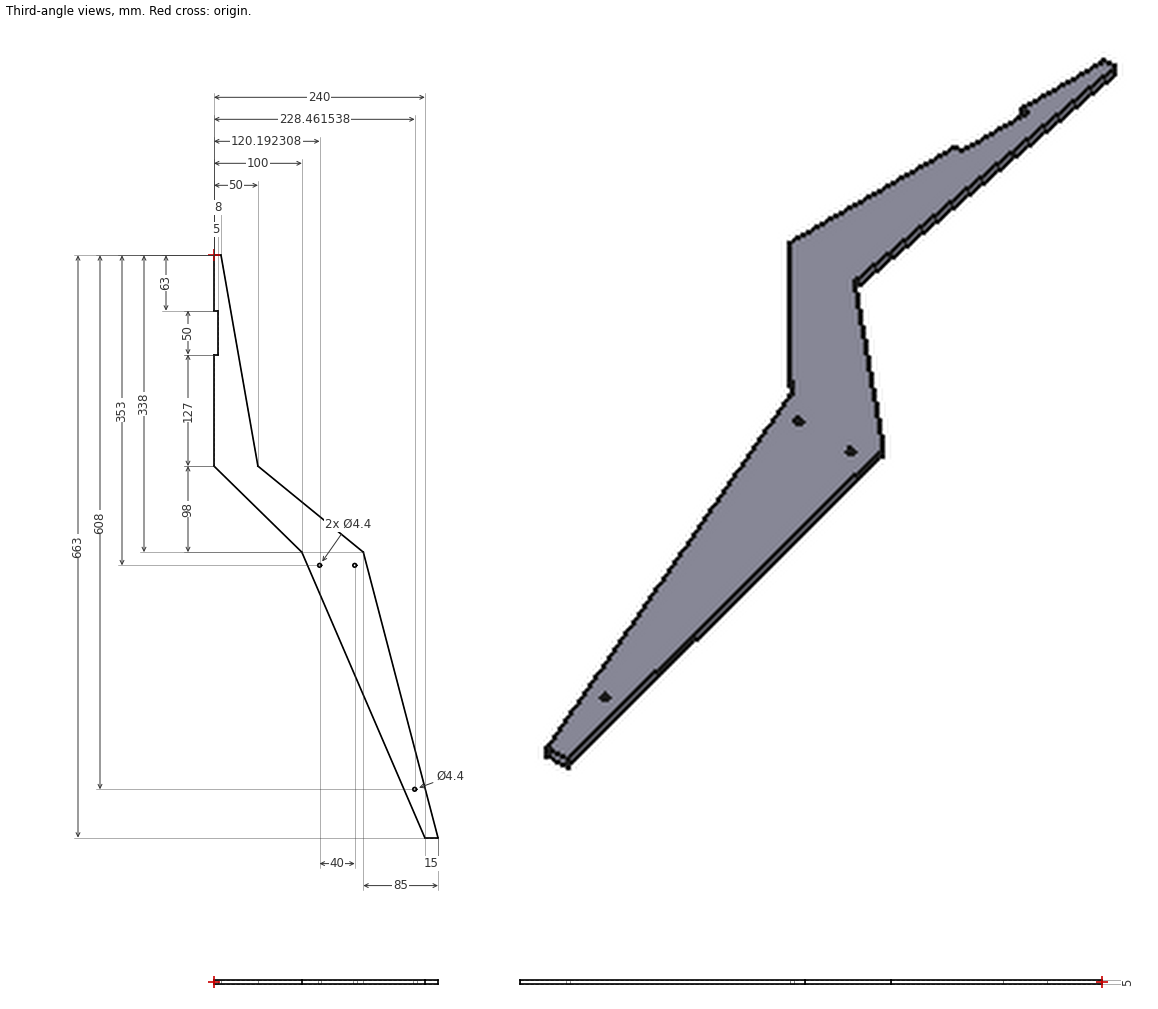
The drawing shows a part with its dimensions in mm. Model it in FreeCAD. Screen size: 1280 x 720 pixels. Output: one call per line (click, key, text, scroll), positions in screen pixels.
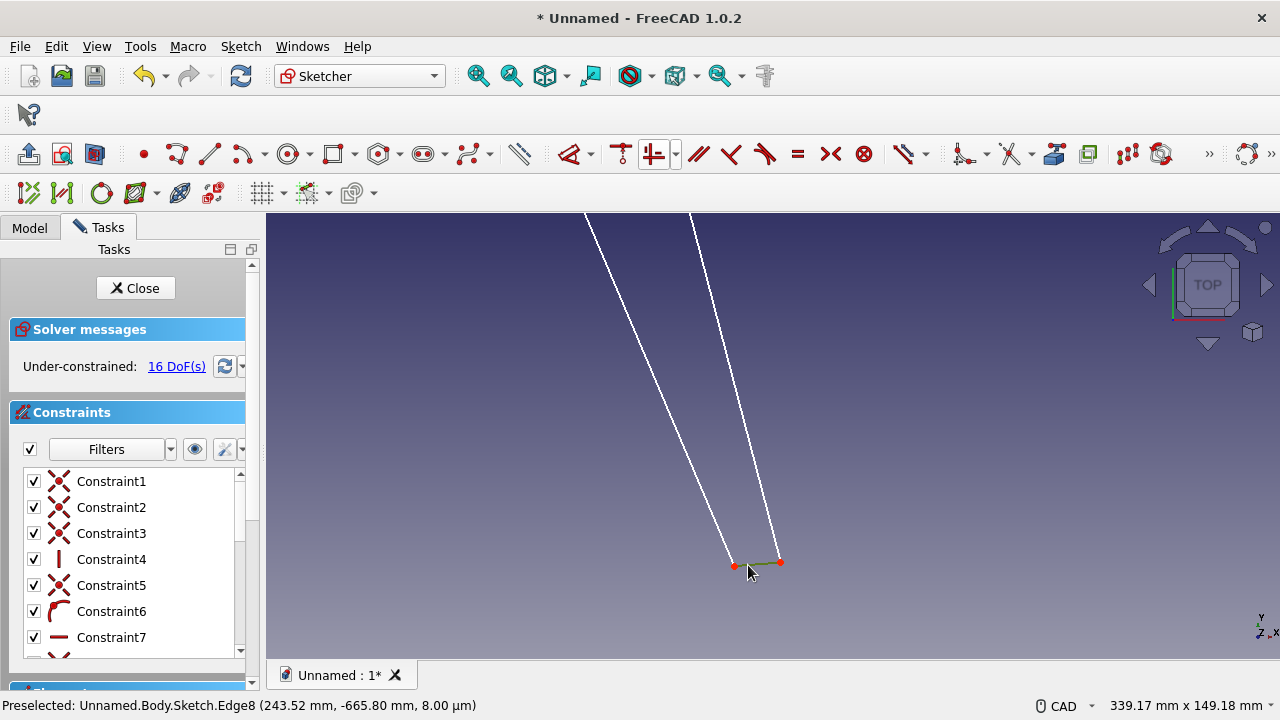
key(h)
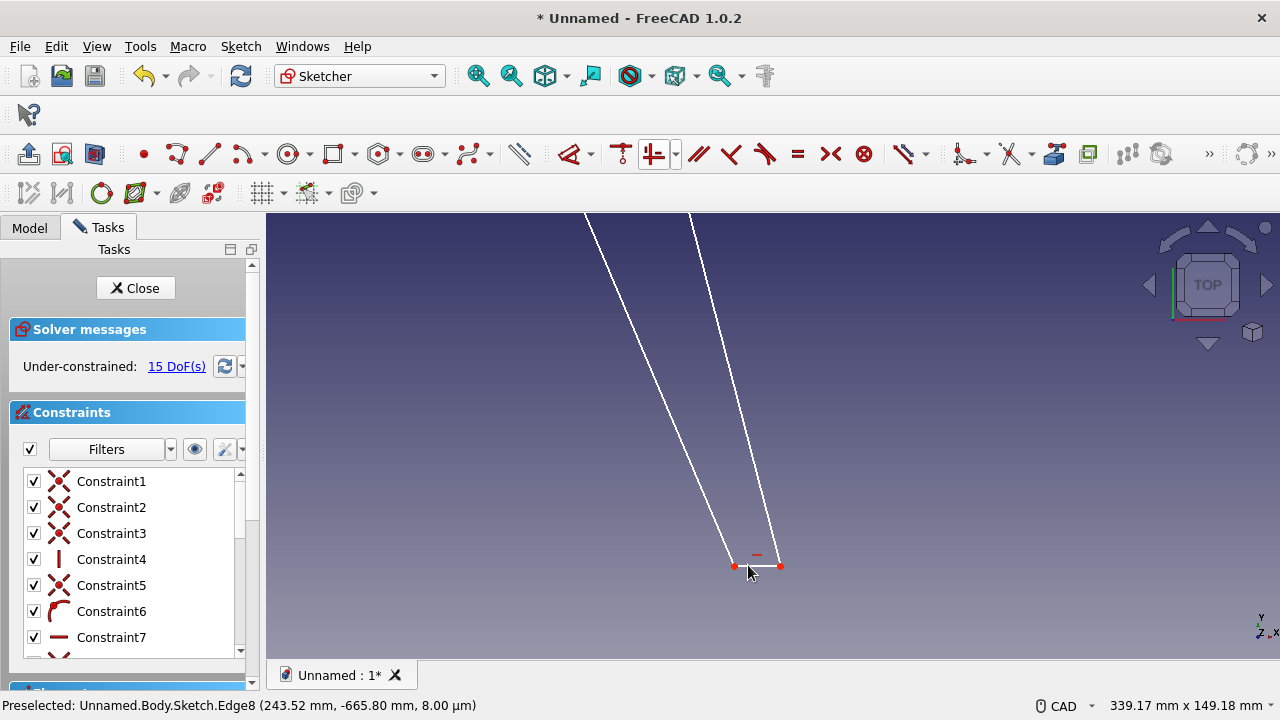
scroll(752, 572, down, 10)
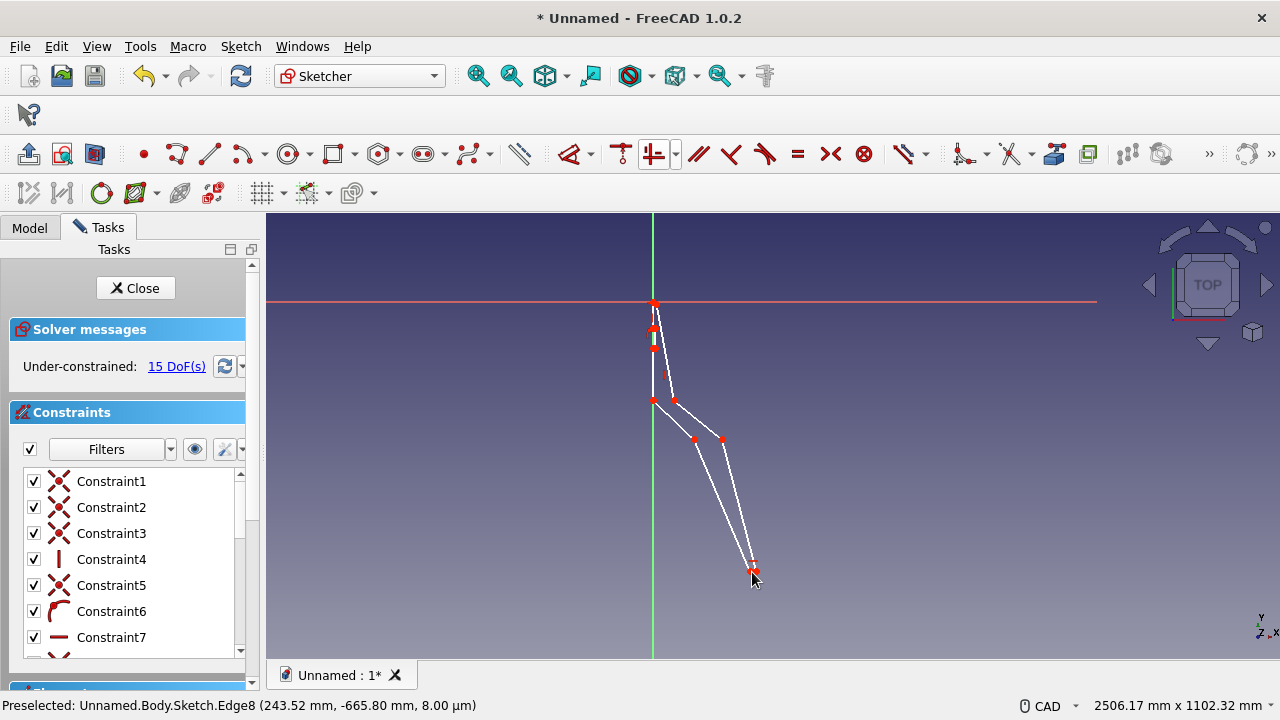
scroll(655, 304, up, 12)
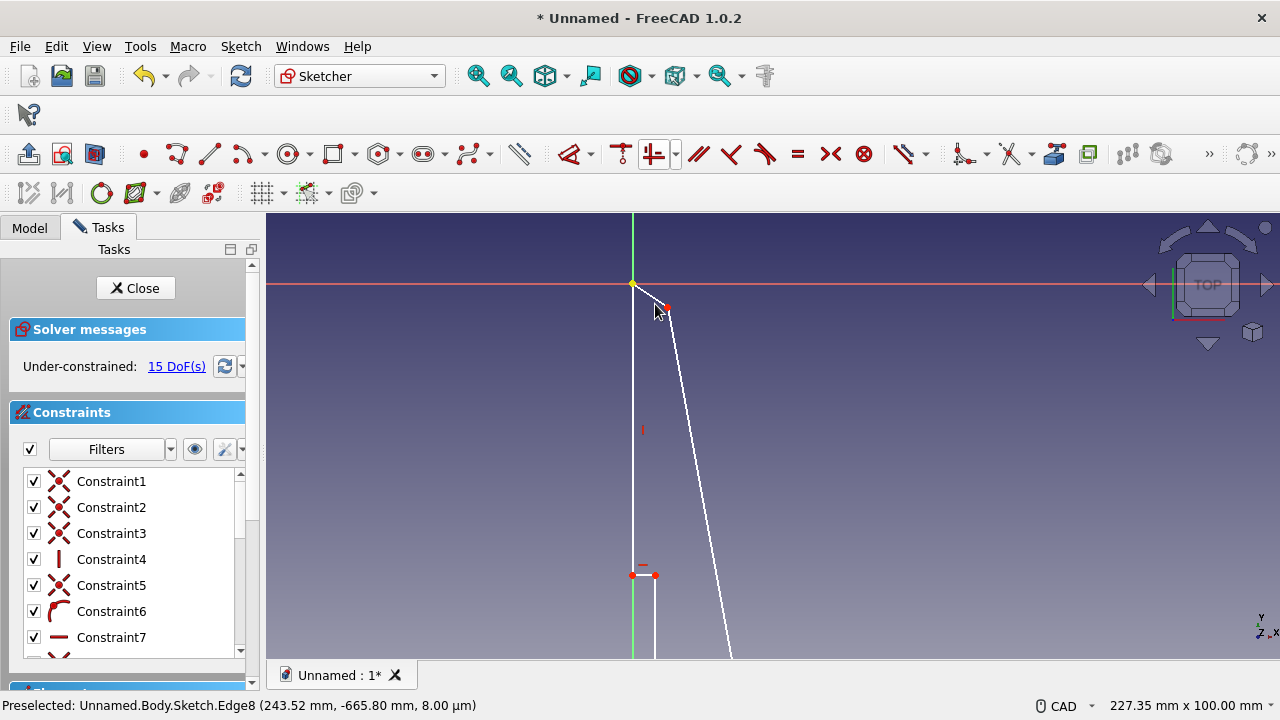
click(654, 298)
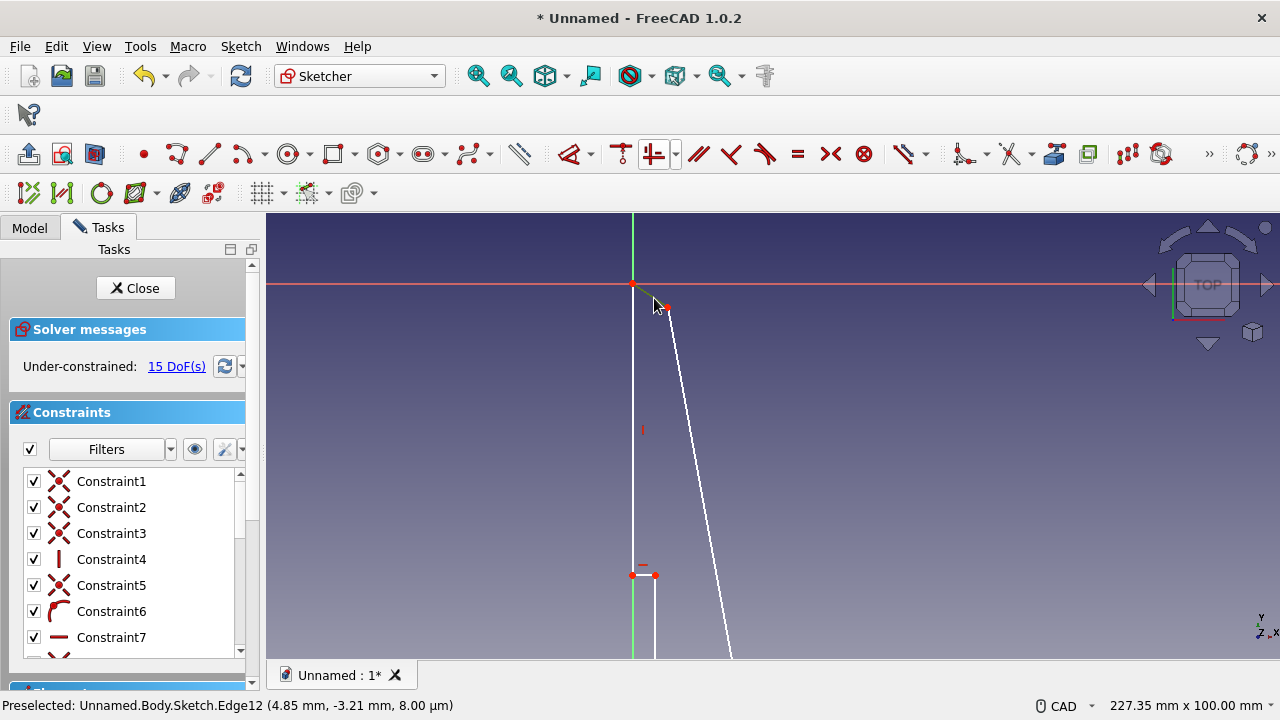
click(676, 154)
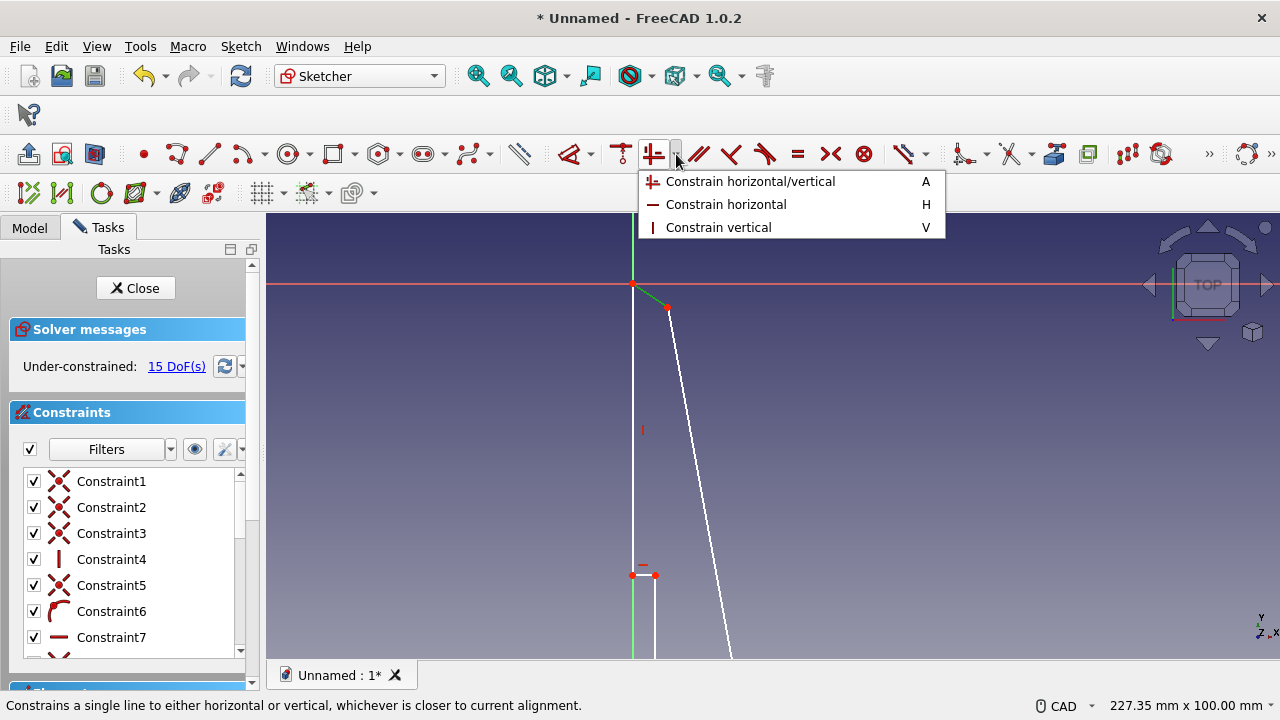
click(792, 204)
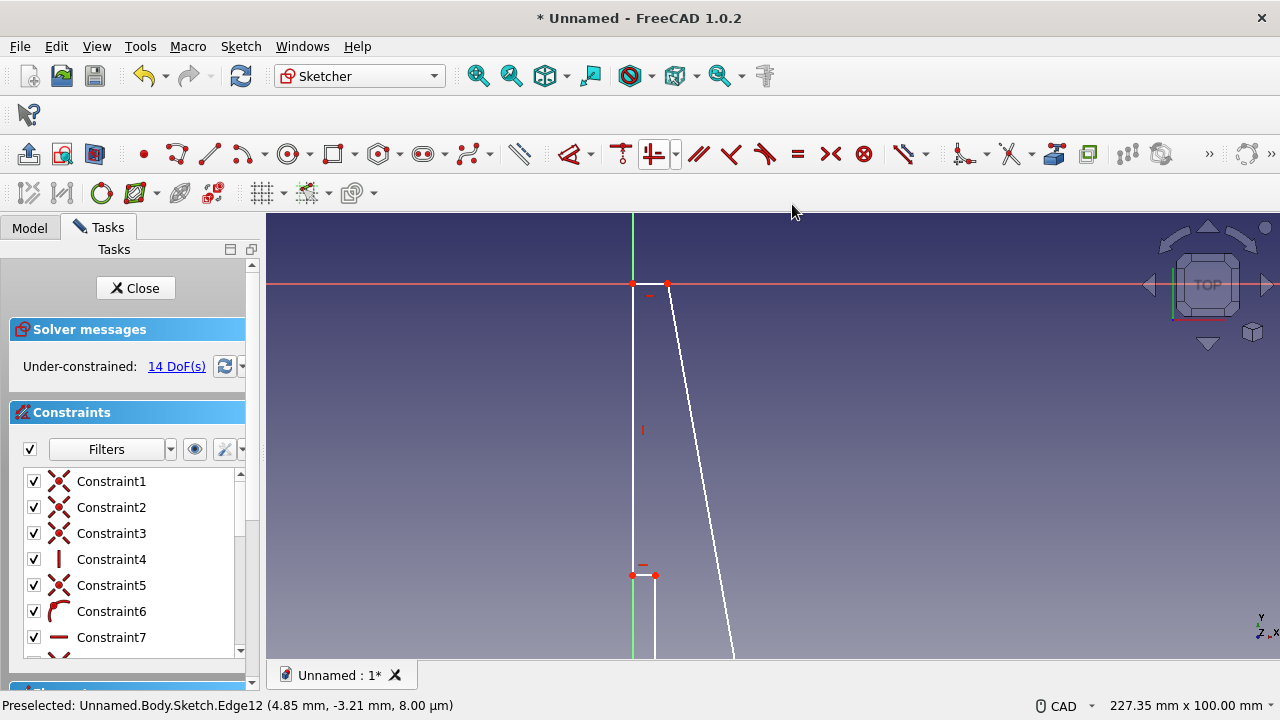
click(568, 154)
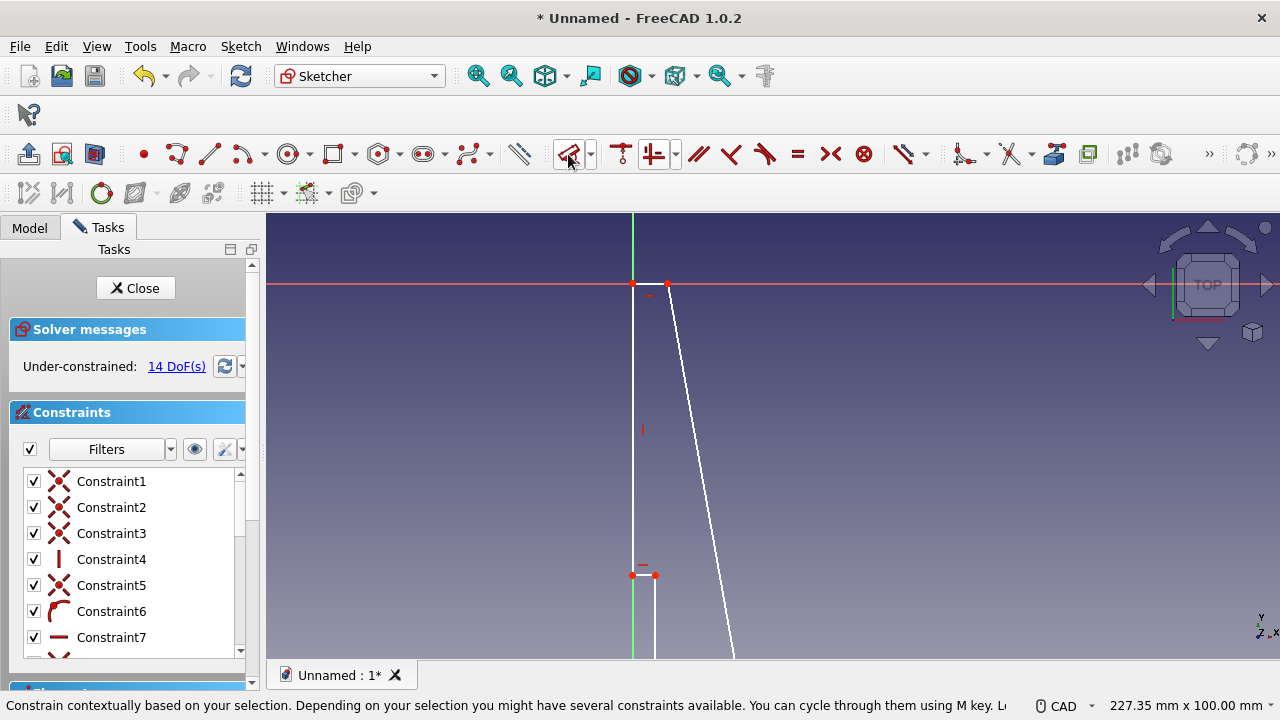
scroll(644, 575, up, 3)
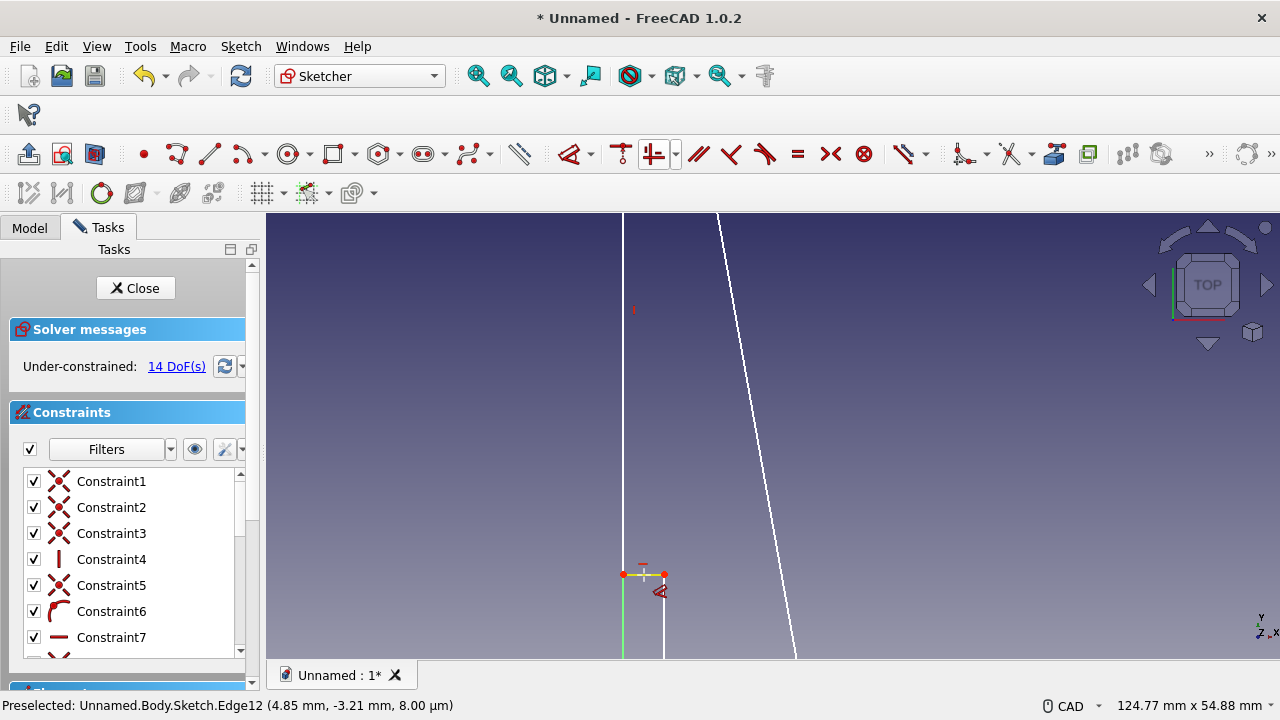
click(644, 575)
click(644, 541)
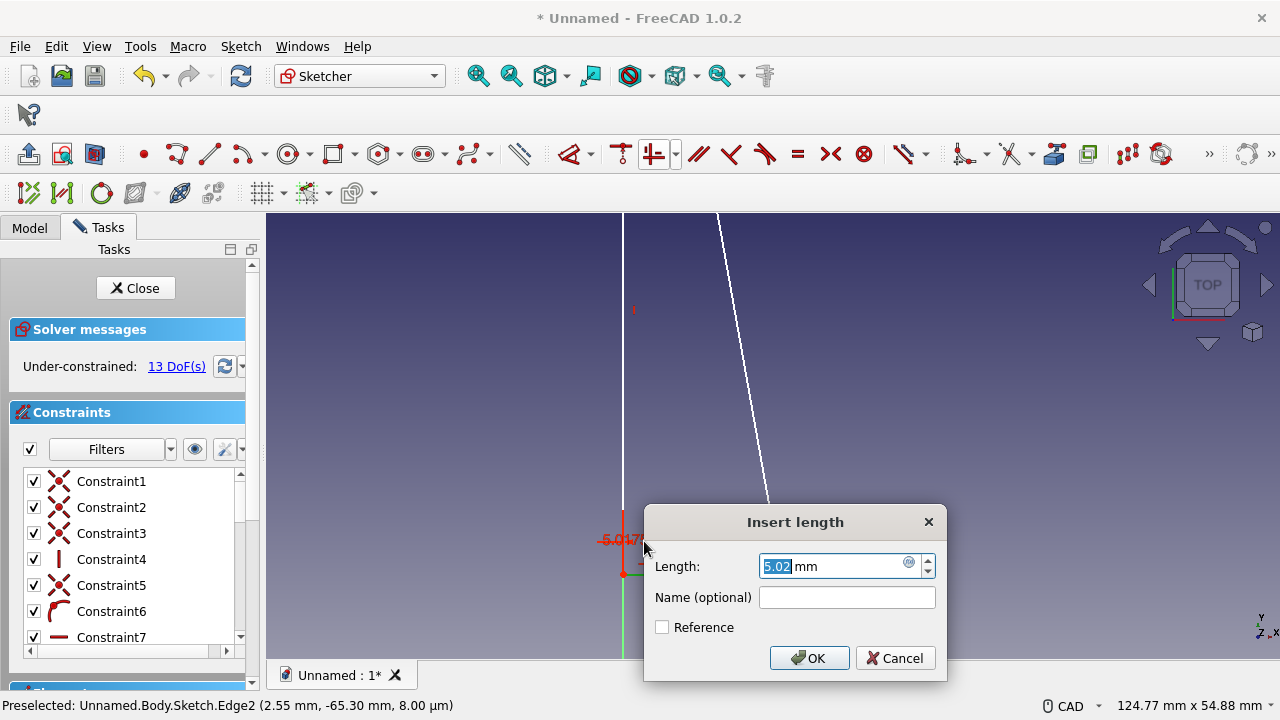
text(5)
key(Return)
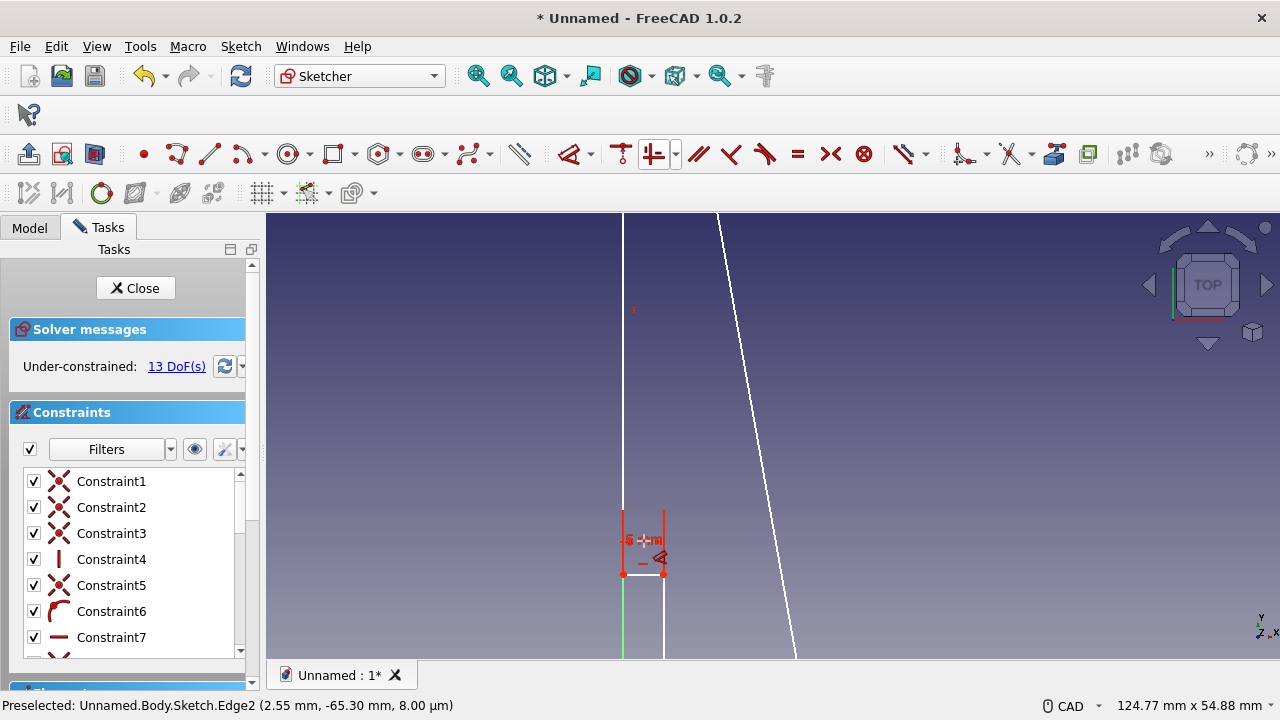
scroll(654, 315, down, 15)